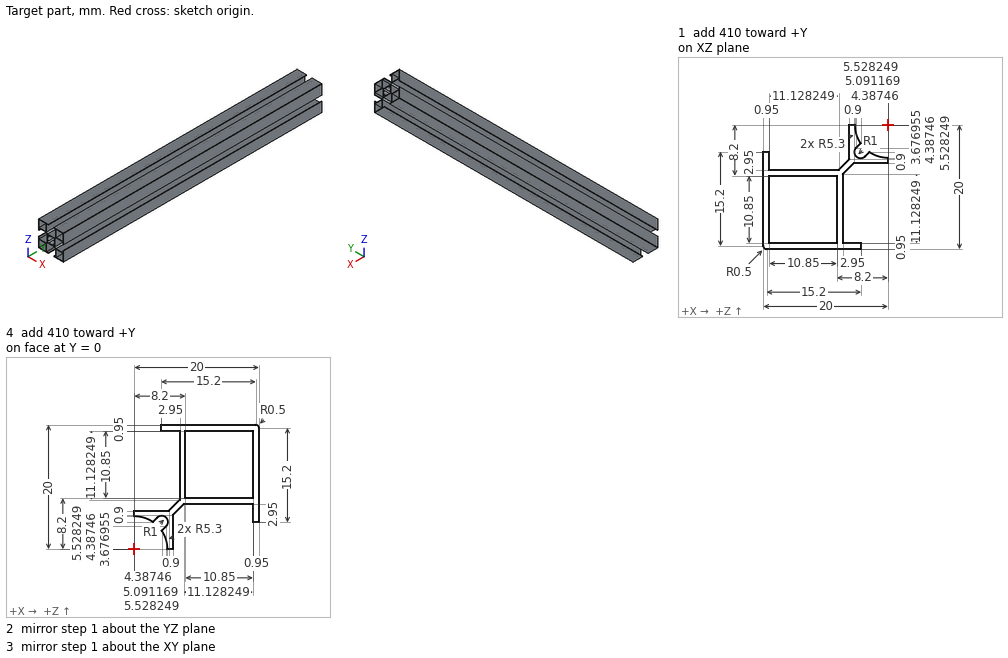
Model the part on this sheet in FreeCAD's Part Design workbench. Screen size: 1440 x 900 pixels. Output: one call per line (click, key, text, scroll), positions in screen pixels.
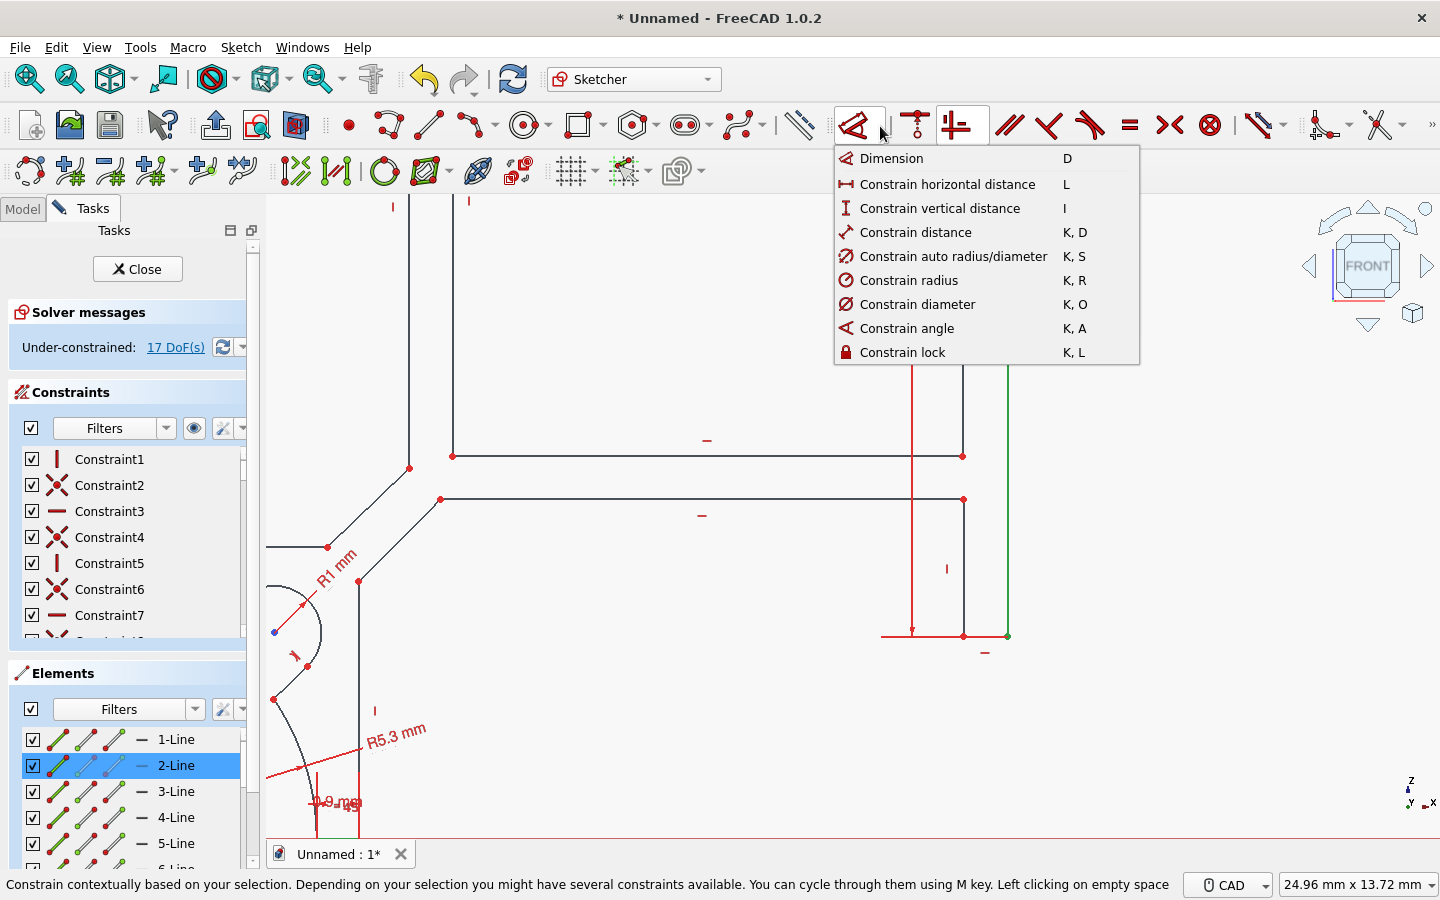
click(987, 184)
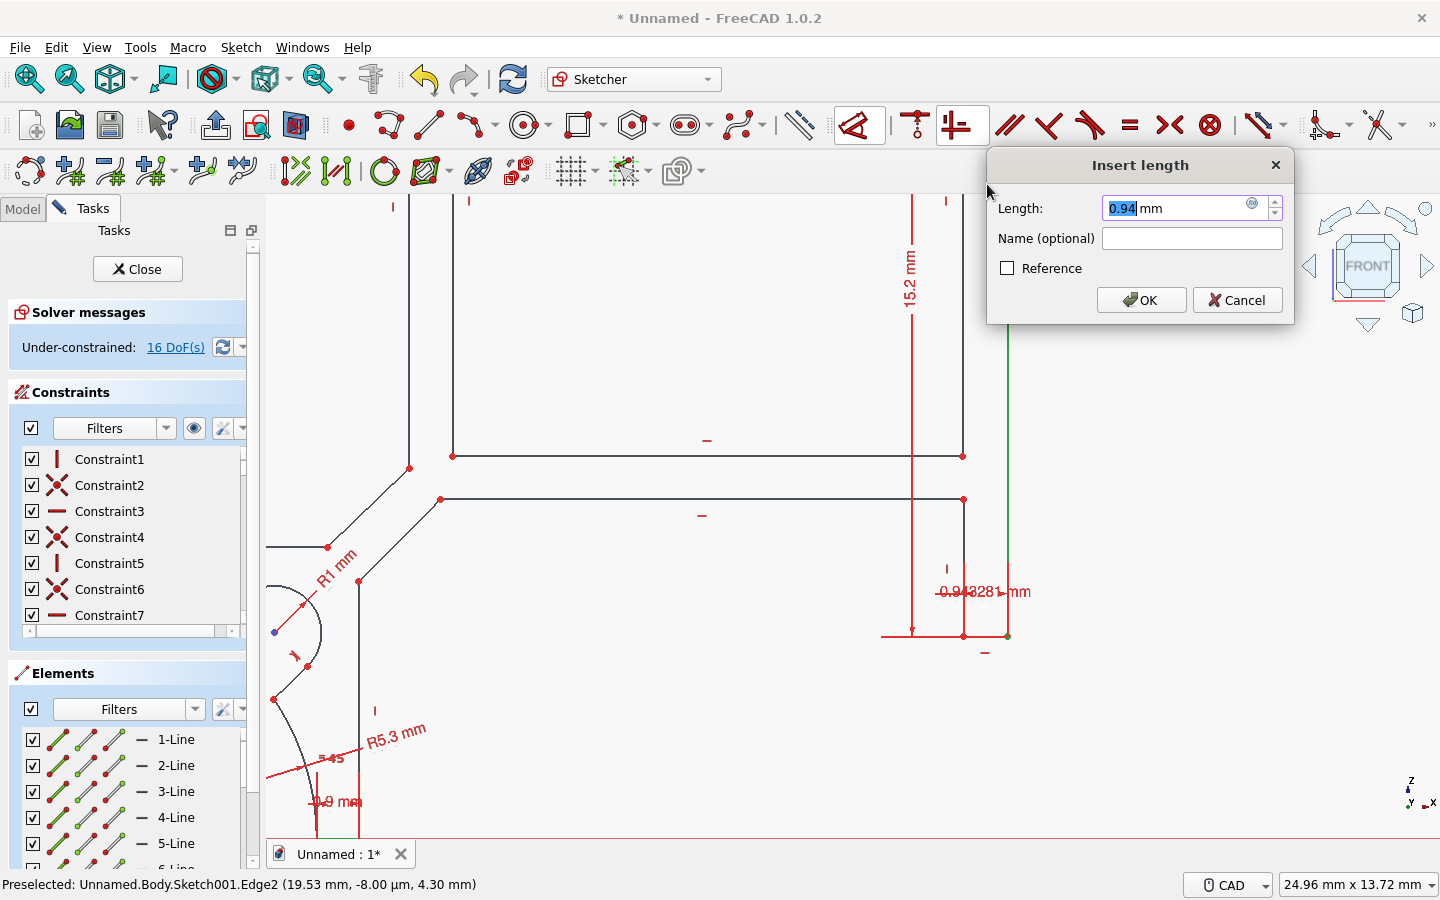
text(0.95)
key(Return)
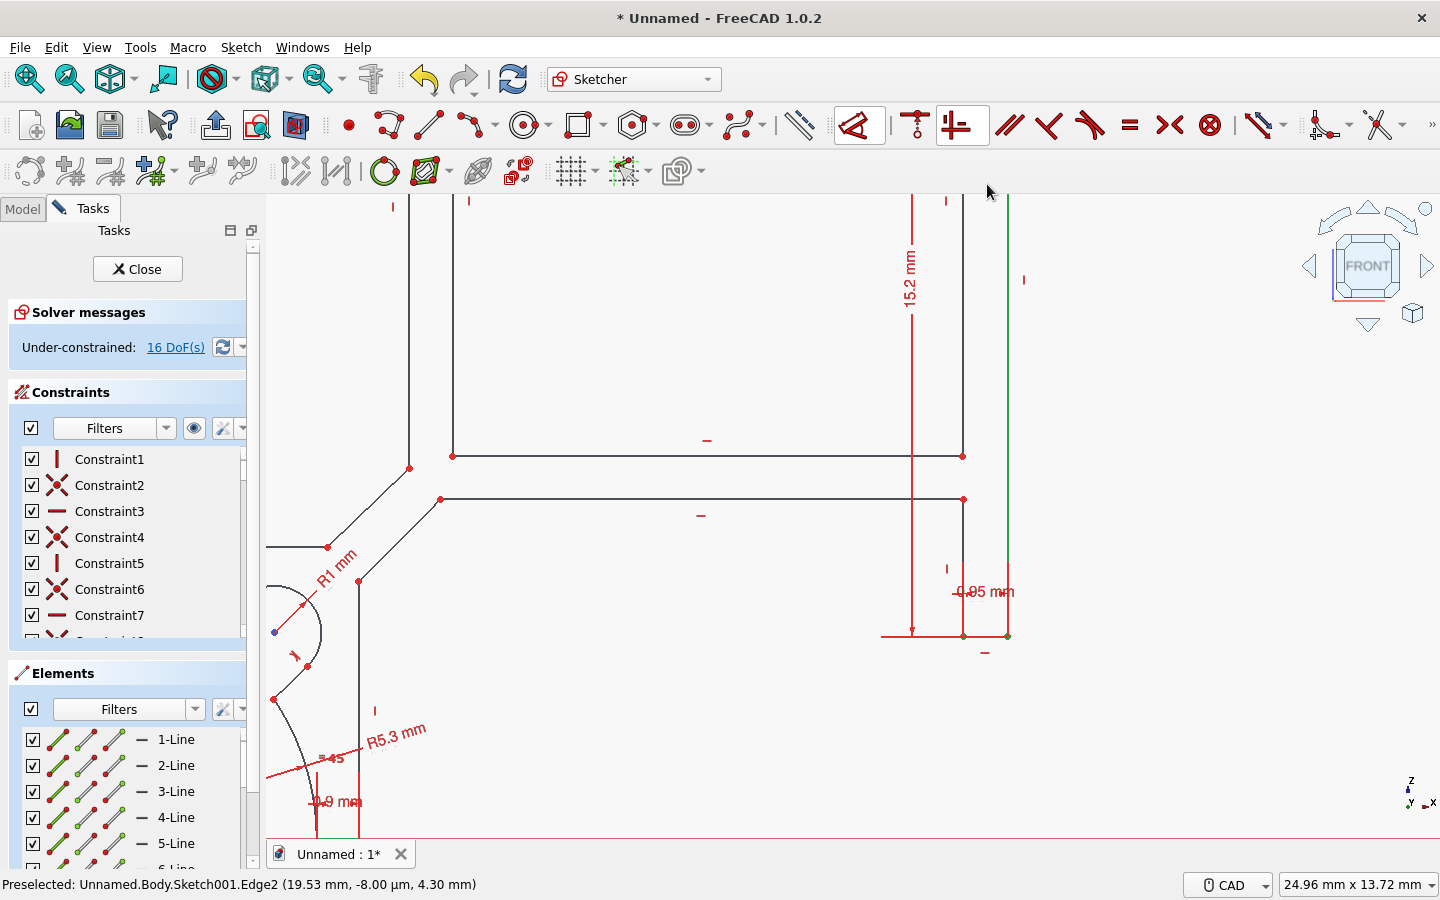
click(963, 541)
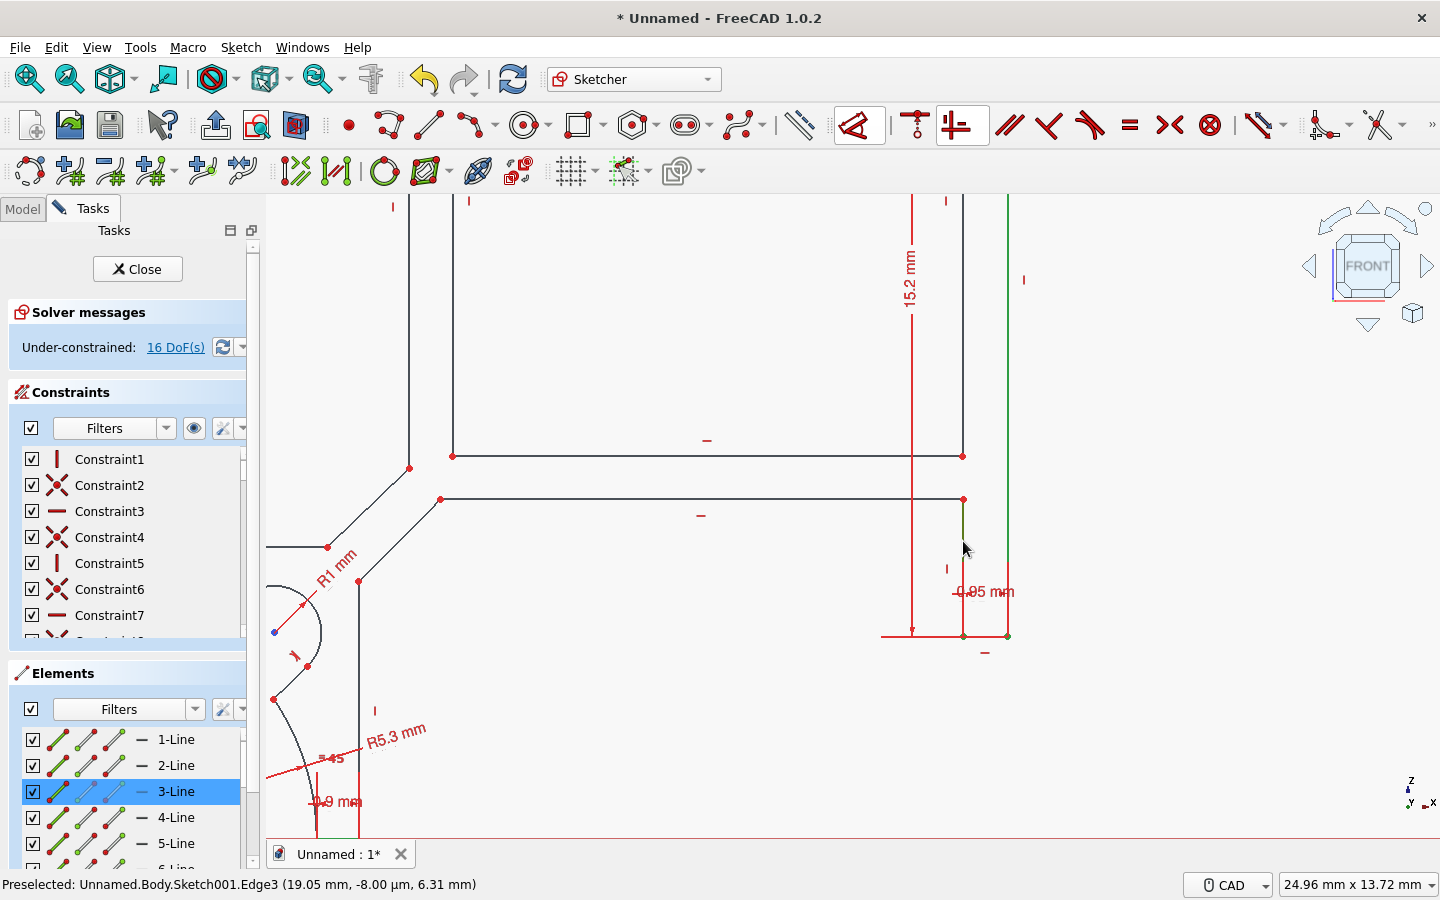
click(880, 126)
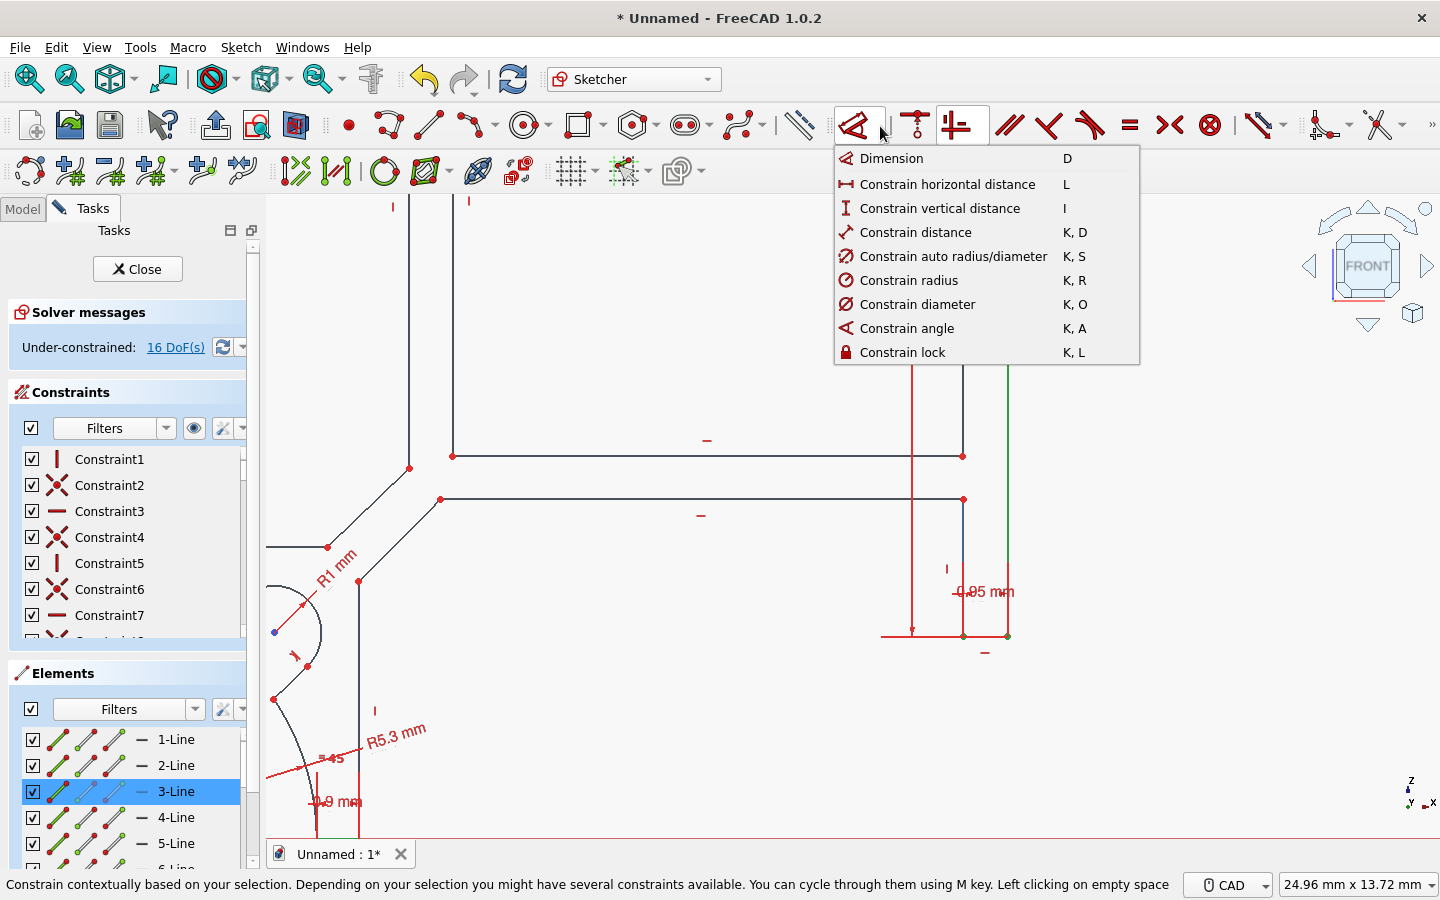
click(987, 208)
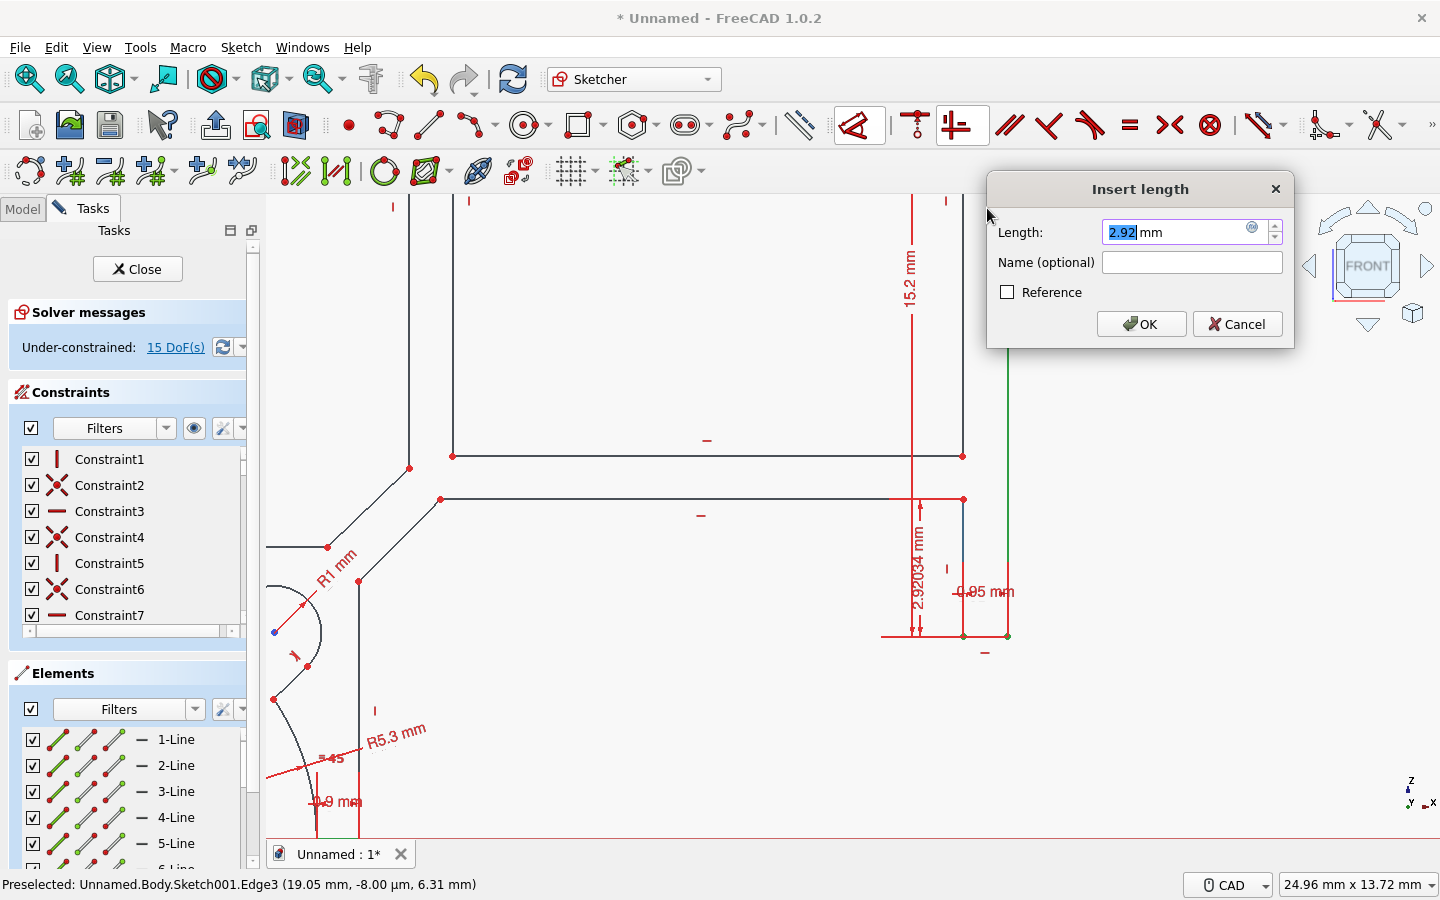
text(2.95)
key(Return)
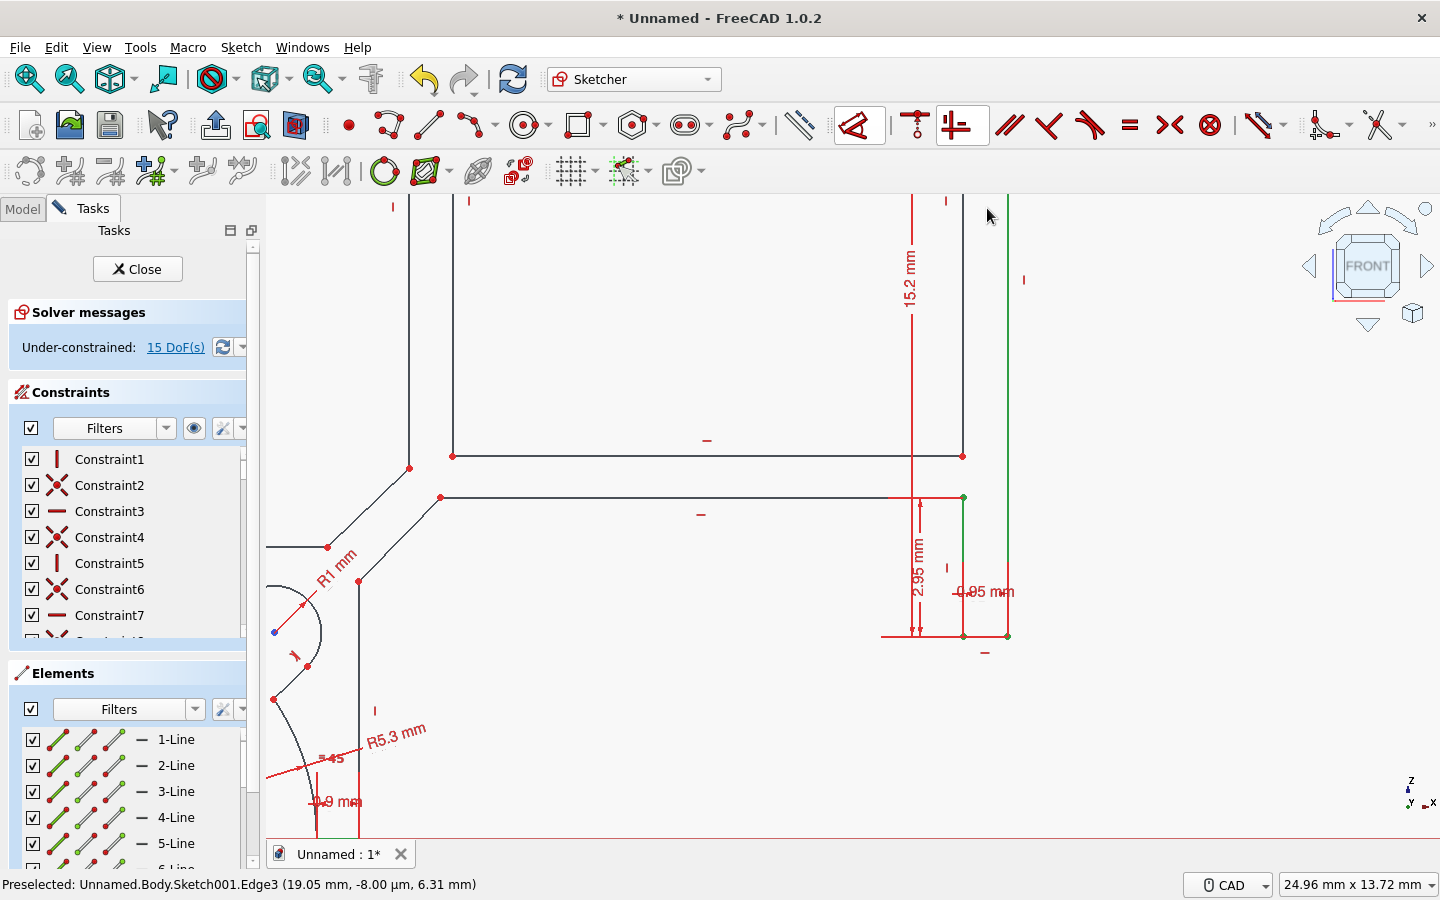
scroll(986, 637, down, 4)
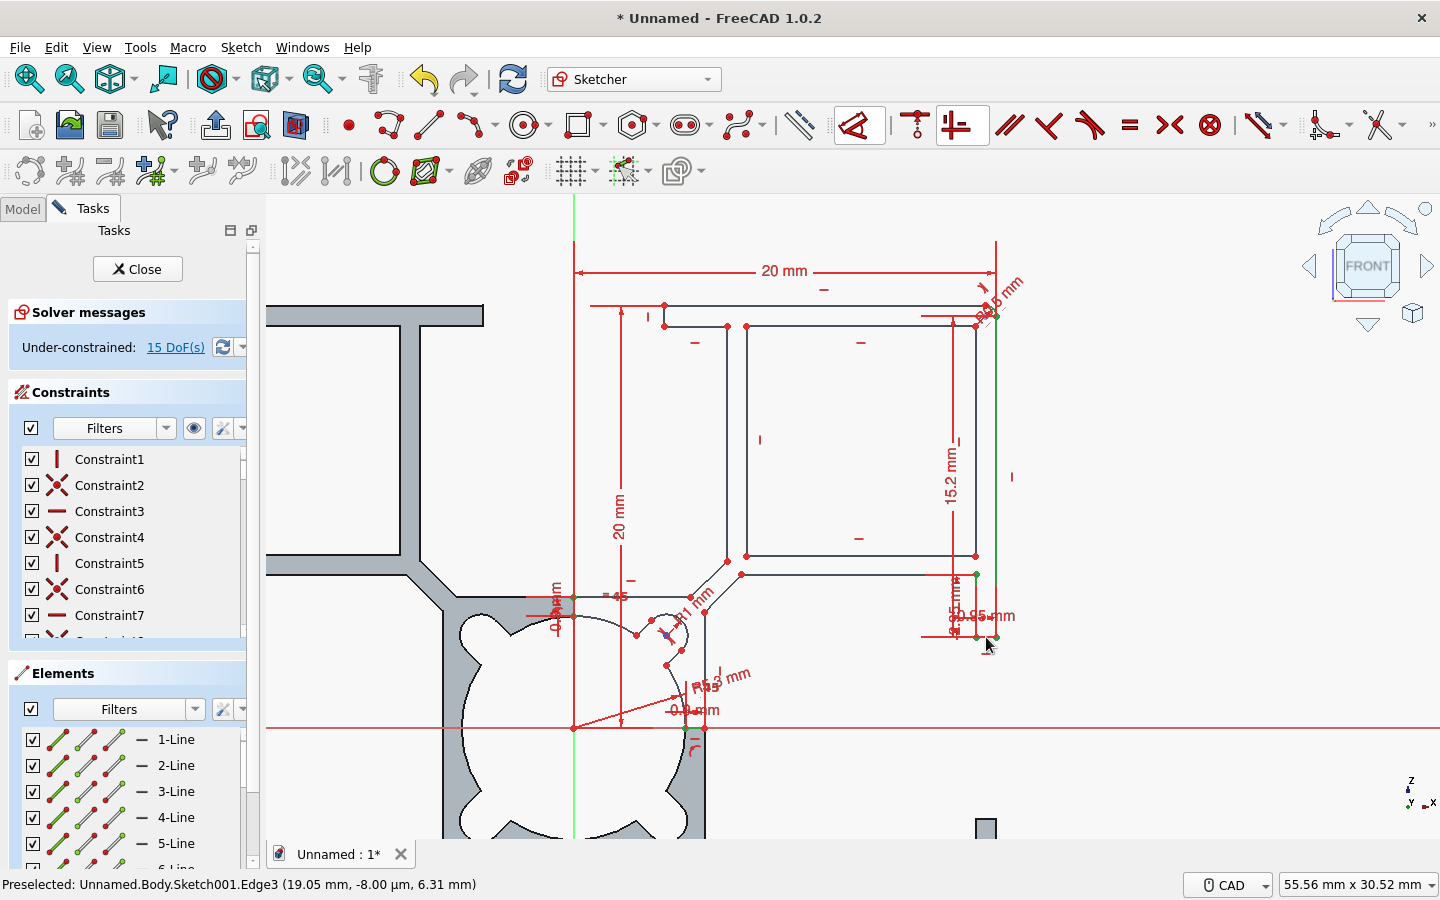
click(708, 327)